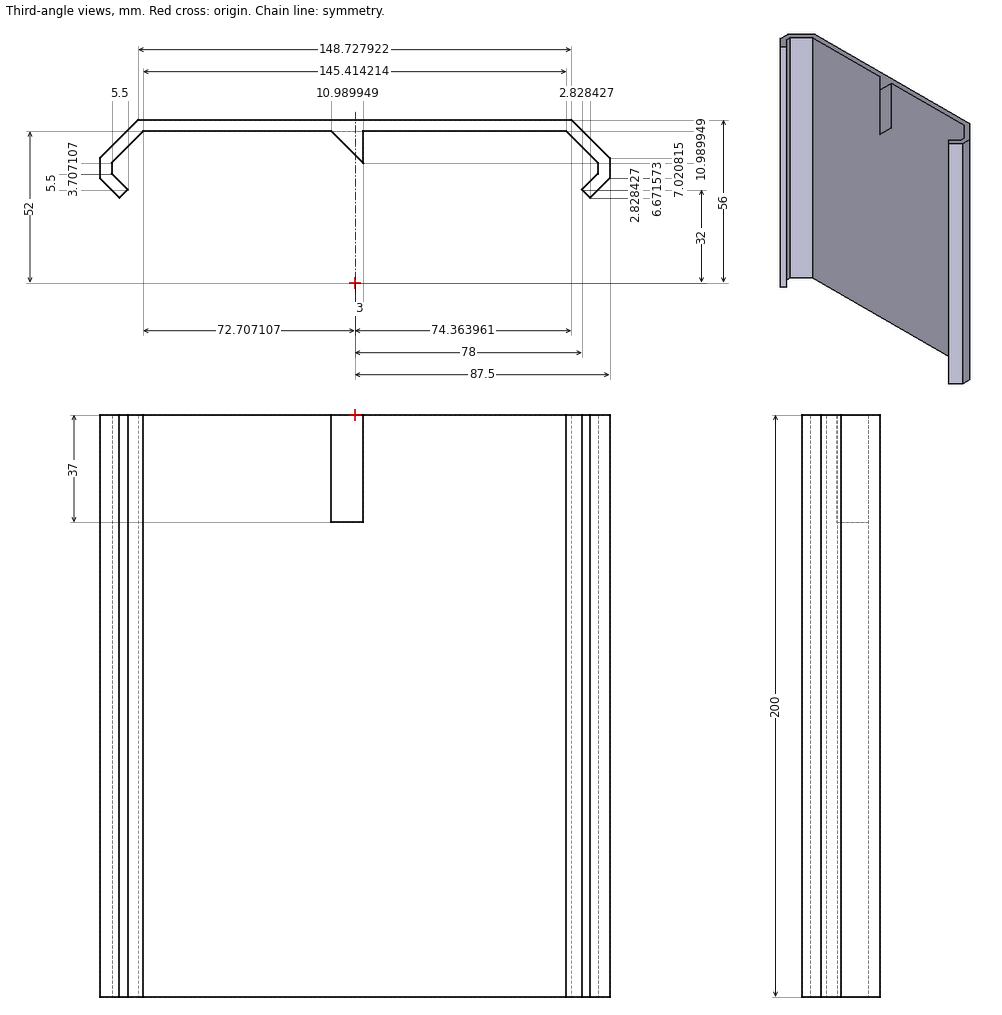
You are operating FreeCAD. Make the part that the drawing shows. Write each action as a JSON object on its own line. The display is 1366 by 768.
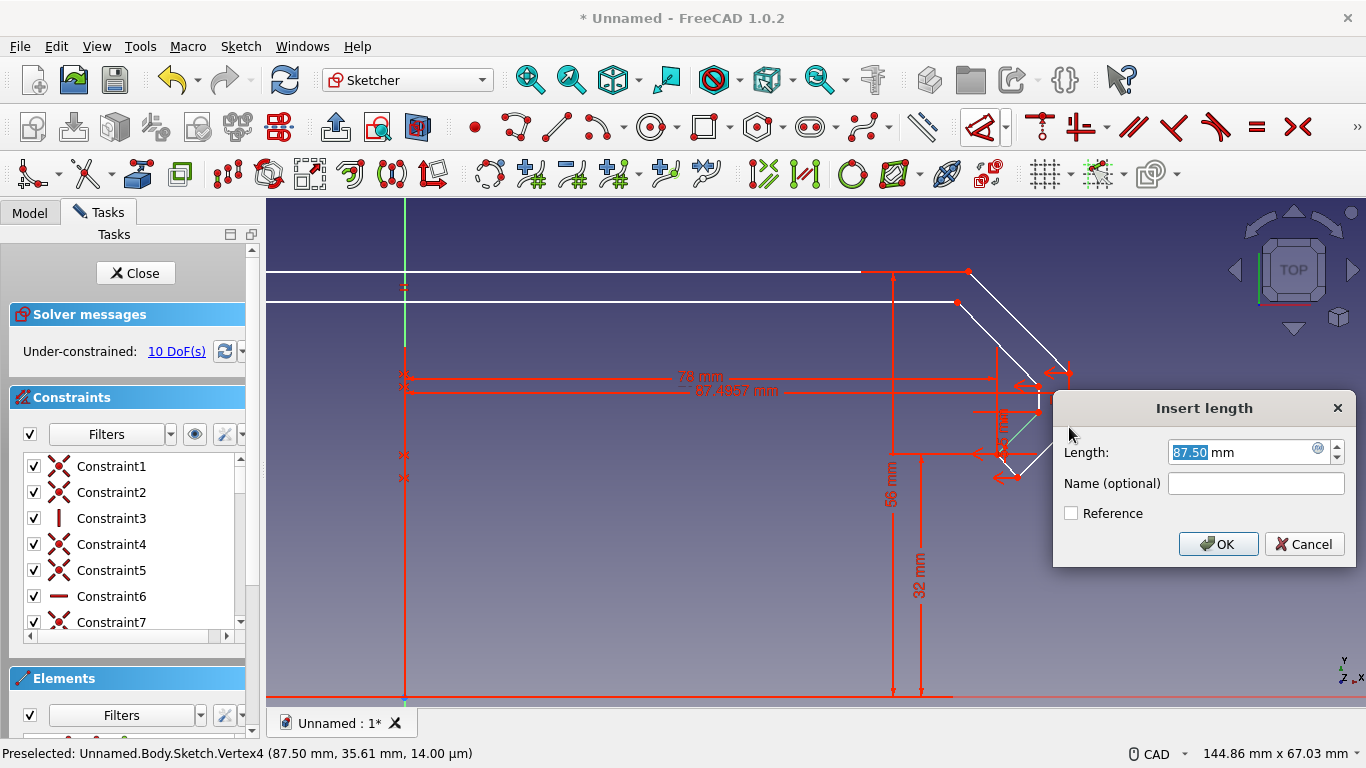
{"action": "type", "text": "87.5"}
{"action": "key", "text": "Return"}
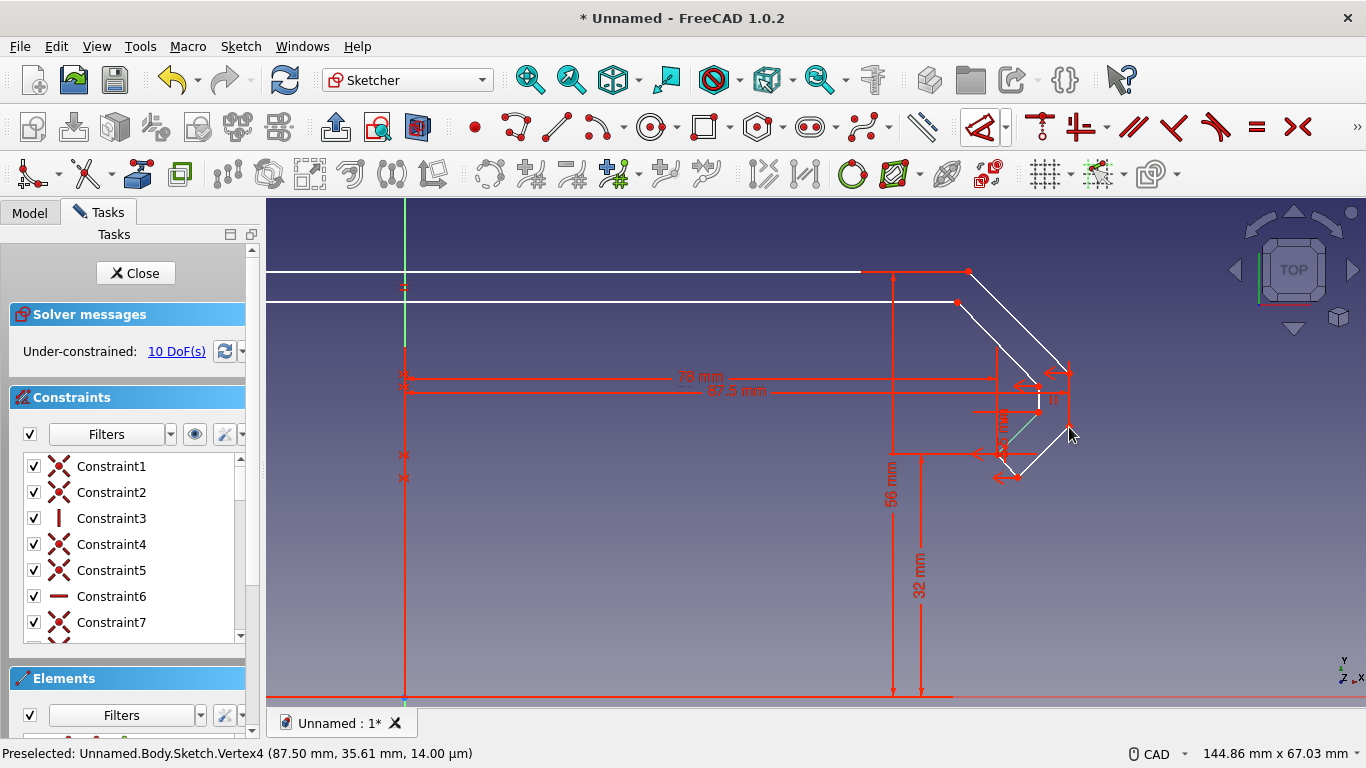
{"action": "left_click", "coordinate": [1069, 411]}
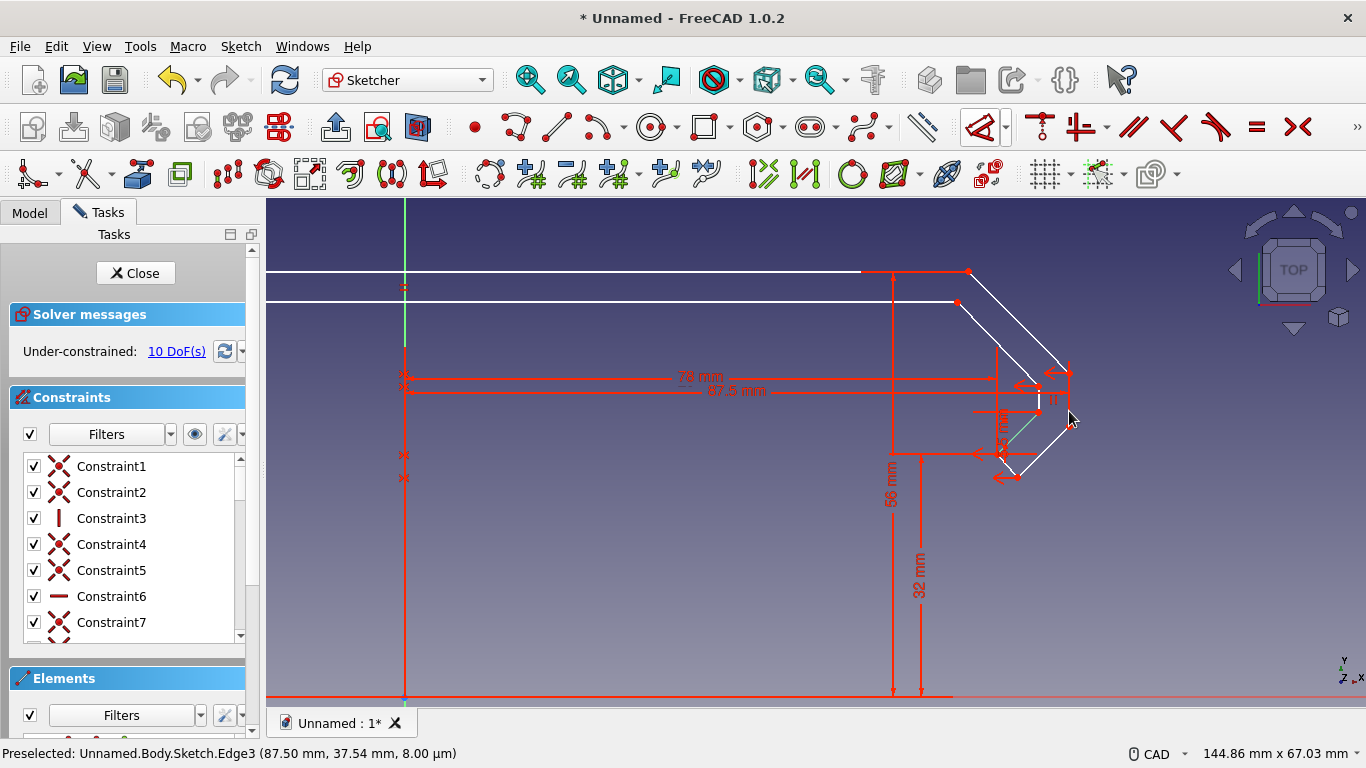
{"action": "left_click", "coordinate": [1006, 128]}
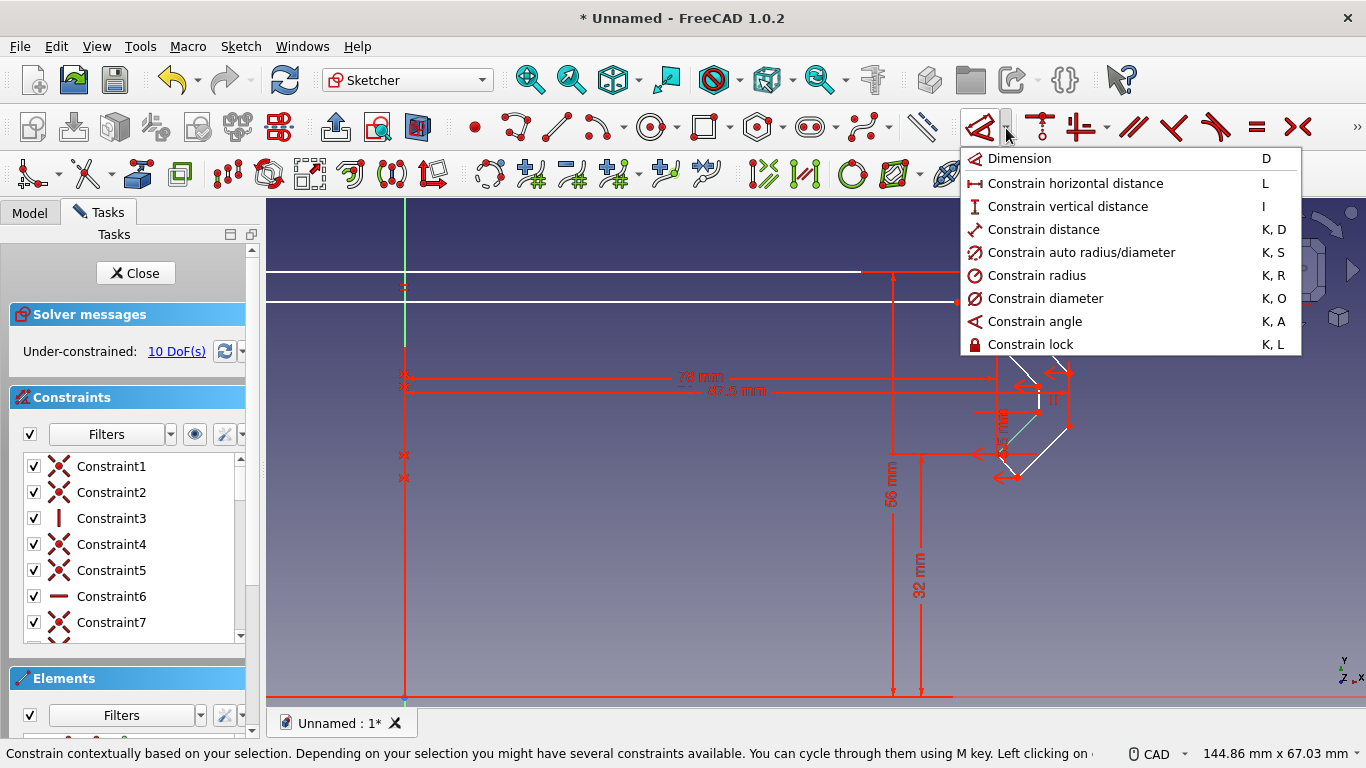
{"action": "left_click", "coordinate": [1131, 206]}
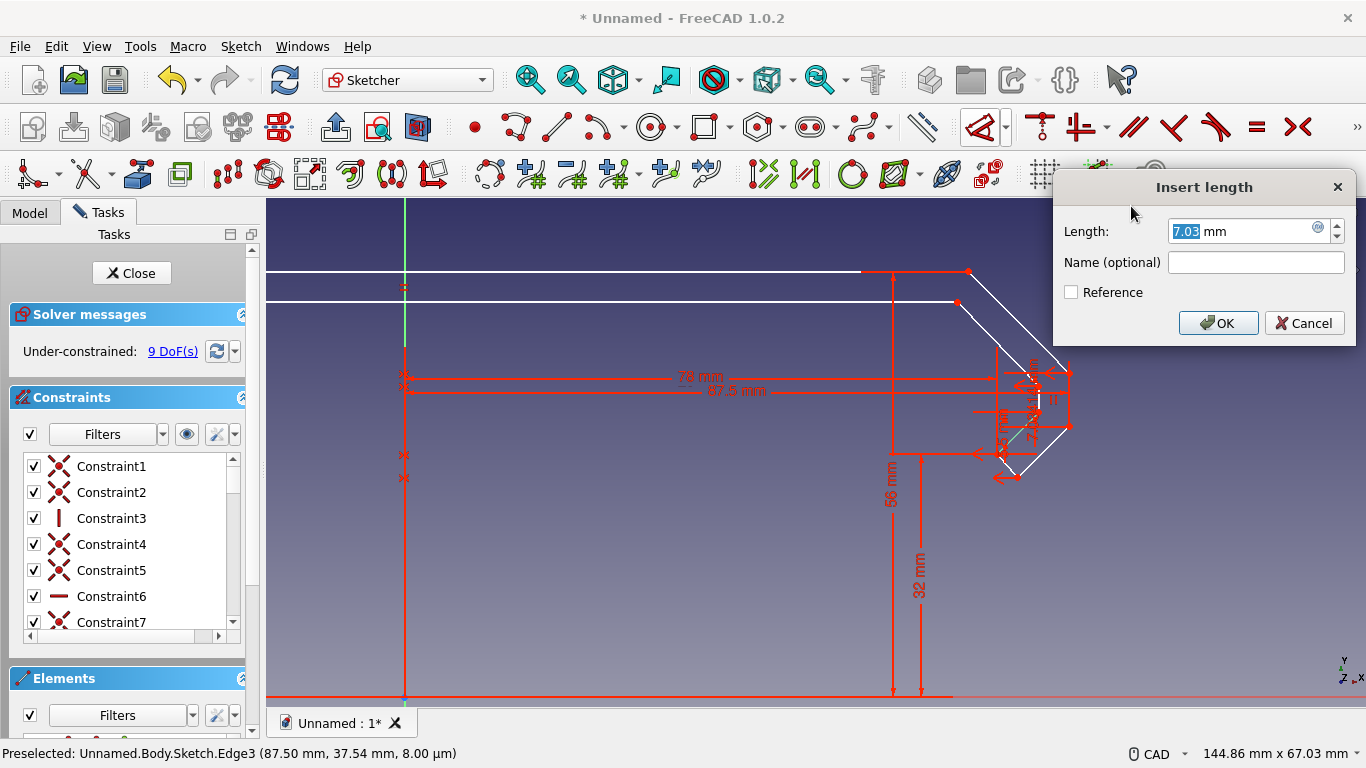
{"action": "type", "text": "7.020815"}
{"action": "key", "text": "Return"}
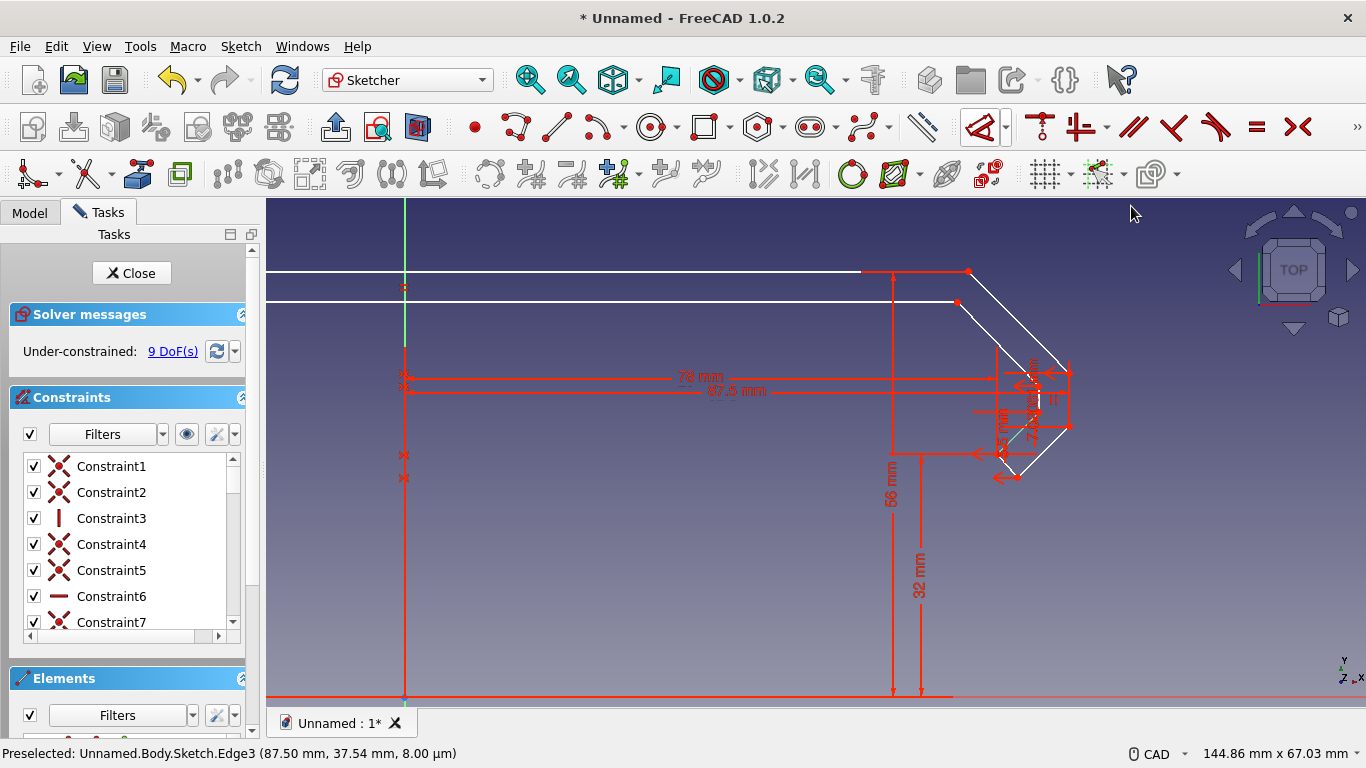
{"action": "scroll", "coordinate": [1027, 426], "scroll_direction": "down", "scroll_amount": 4}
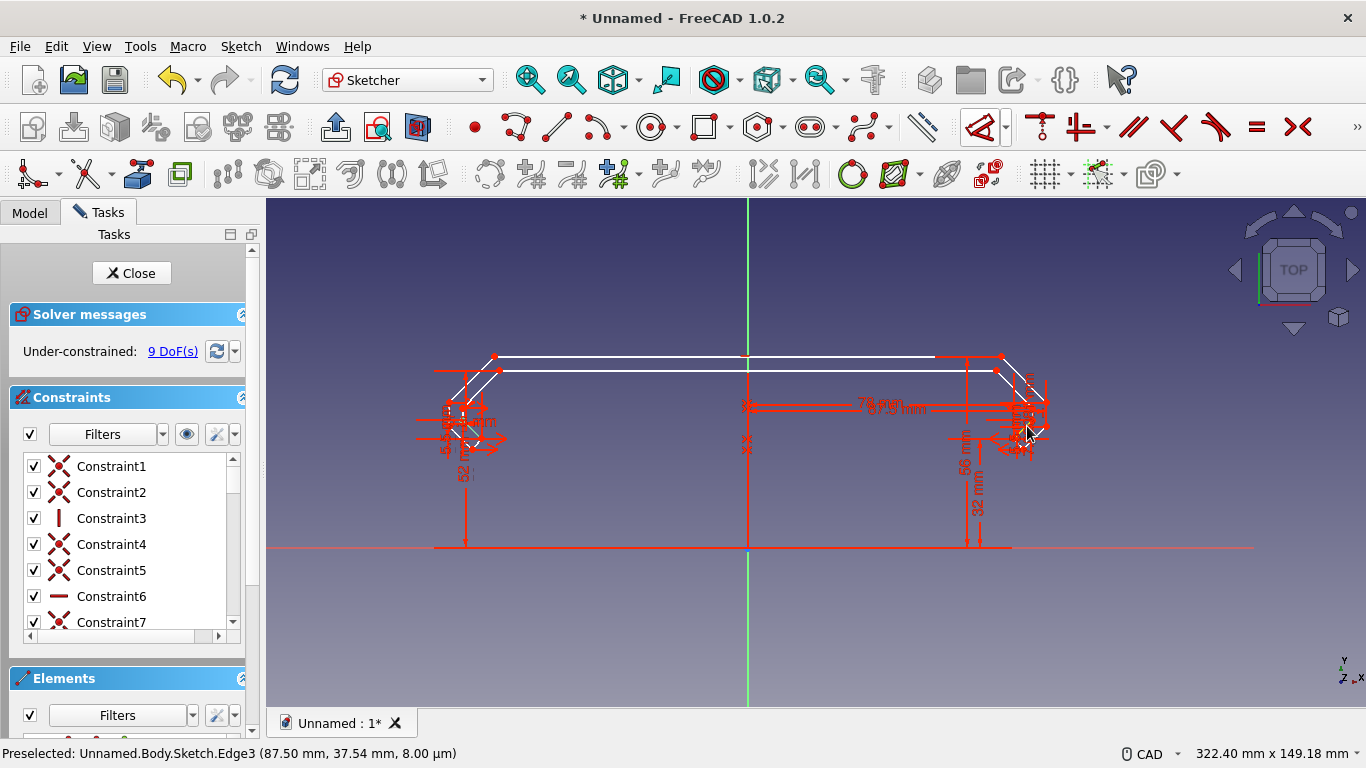
{"action": "scroll", "coordinate": [449, 410], "scroll_direction": "up", "scroll_amount": 4}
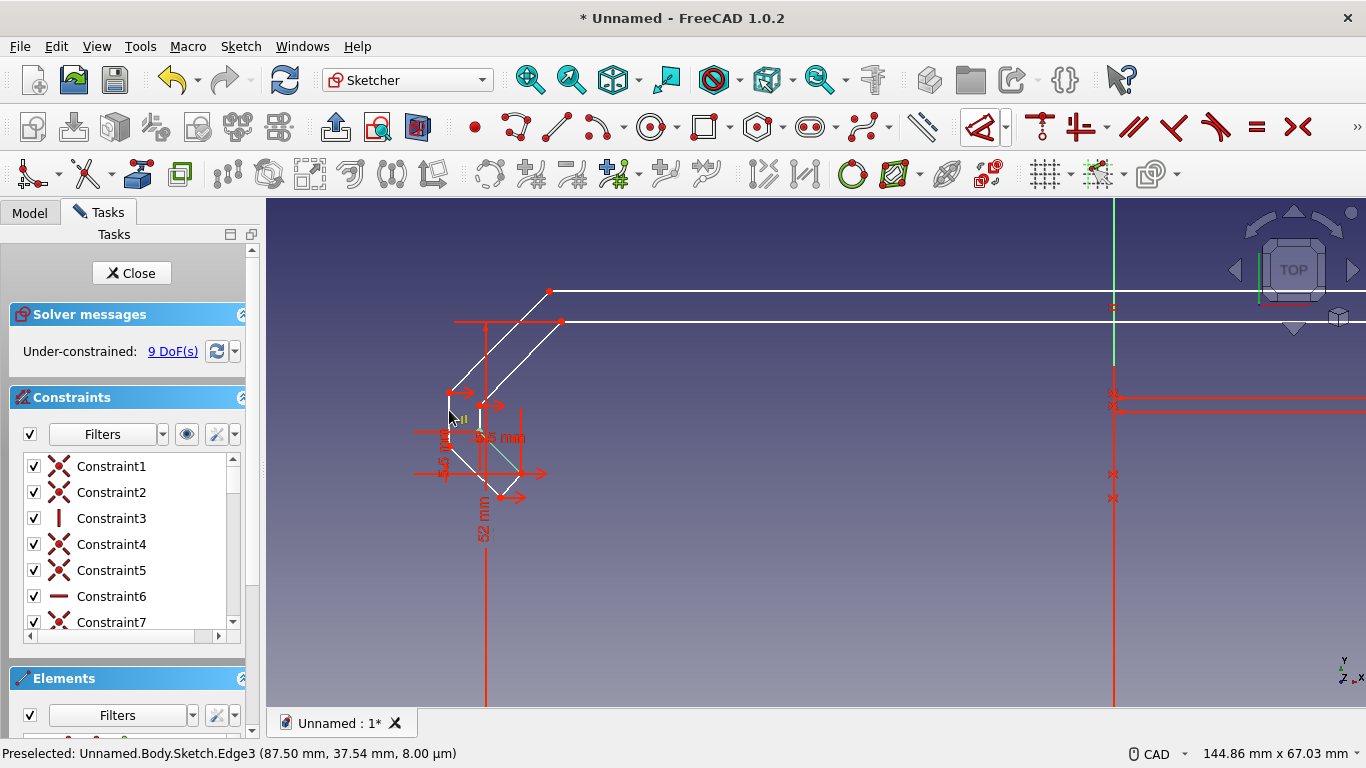
{"action": "left_click", "coordinate": [449, 409]}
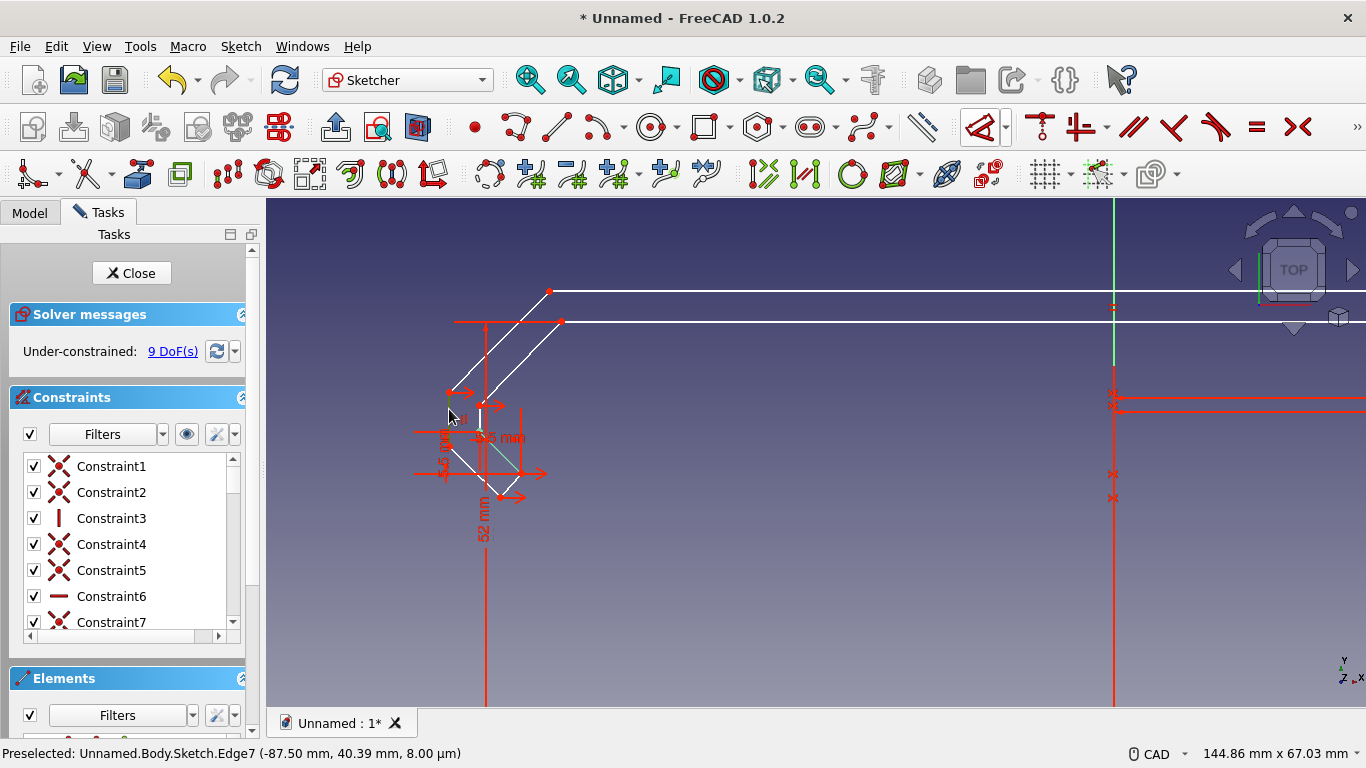
{"action": "key", "text": "i"}